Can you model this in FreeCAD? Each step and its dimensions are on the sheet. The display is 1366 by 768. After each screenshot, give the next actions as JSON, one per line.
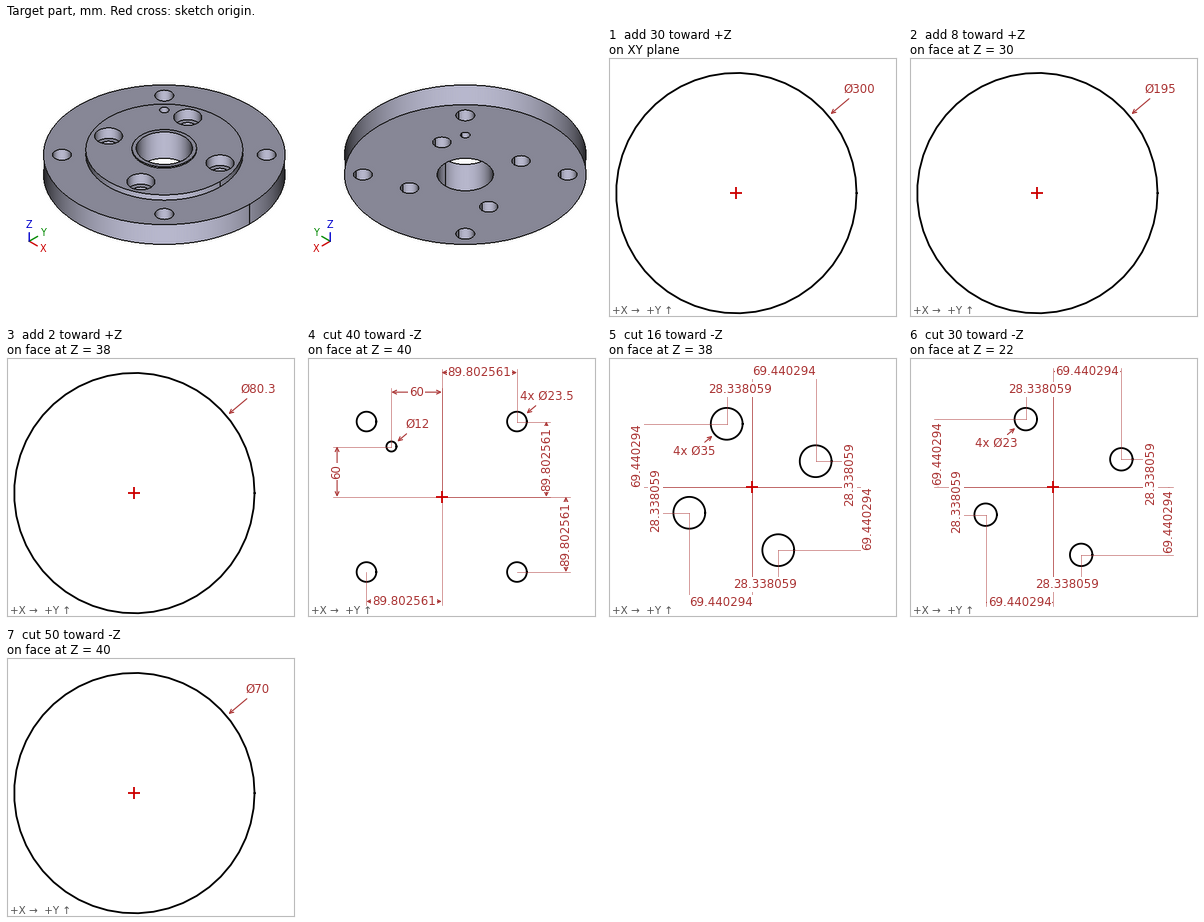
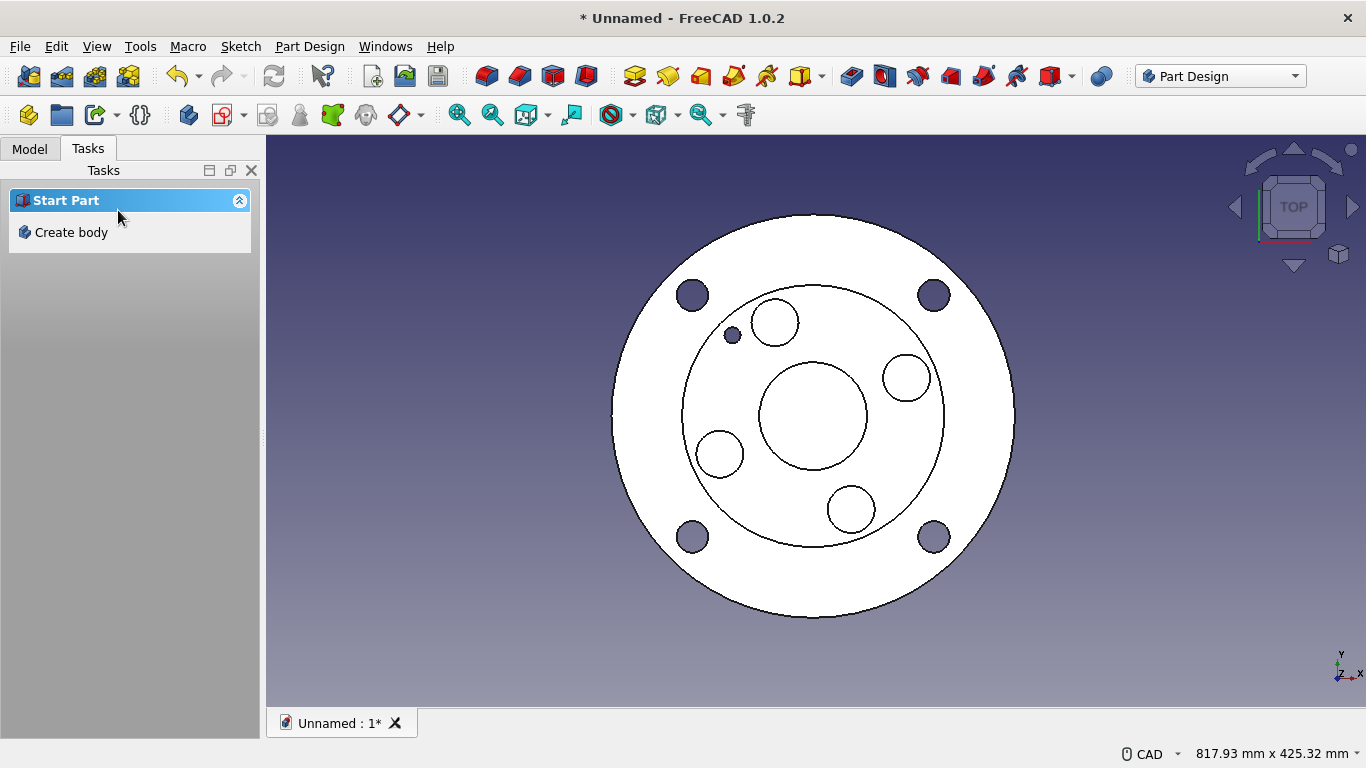
{"action": "left_click", "coordinate": [720, 453]}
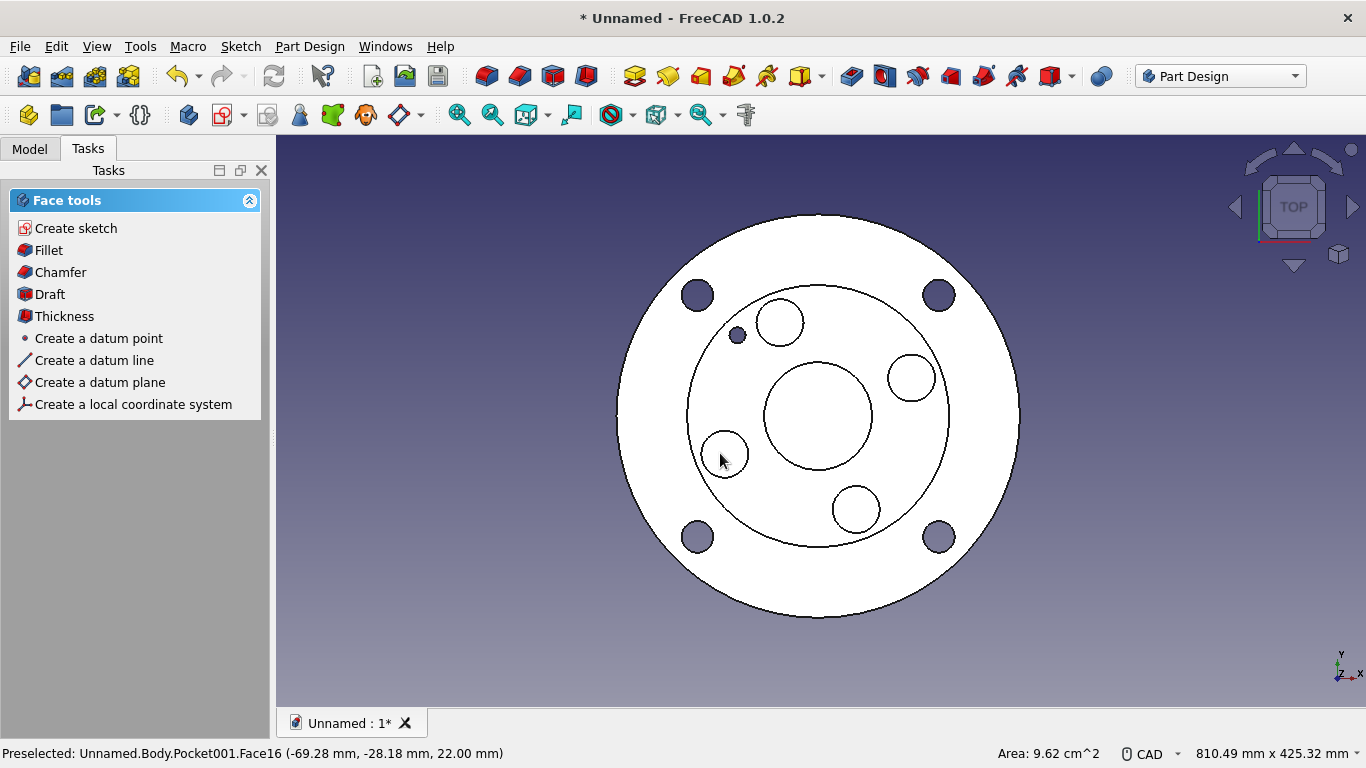
{"action": "left_click", "coordinate": [222, 116]}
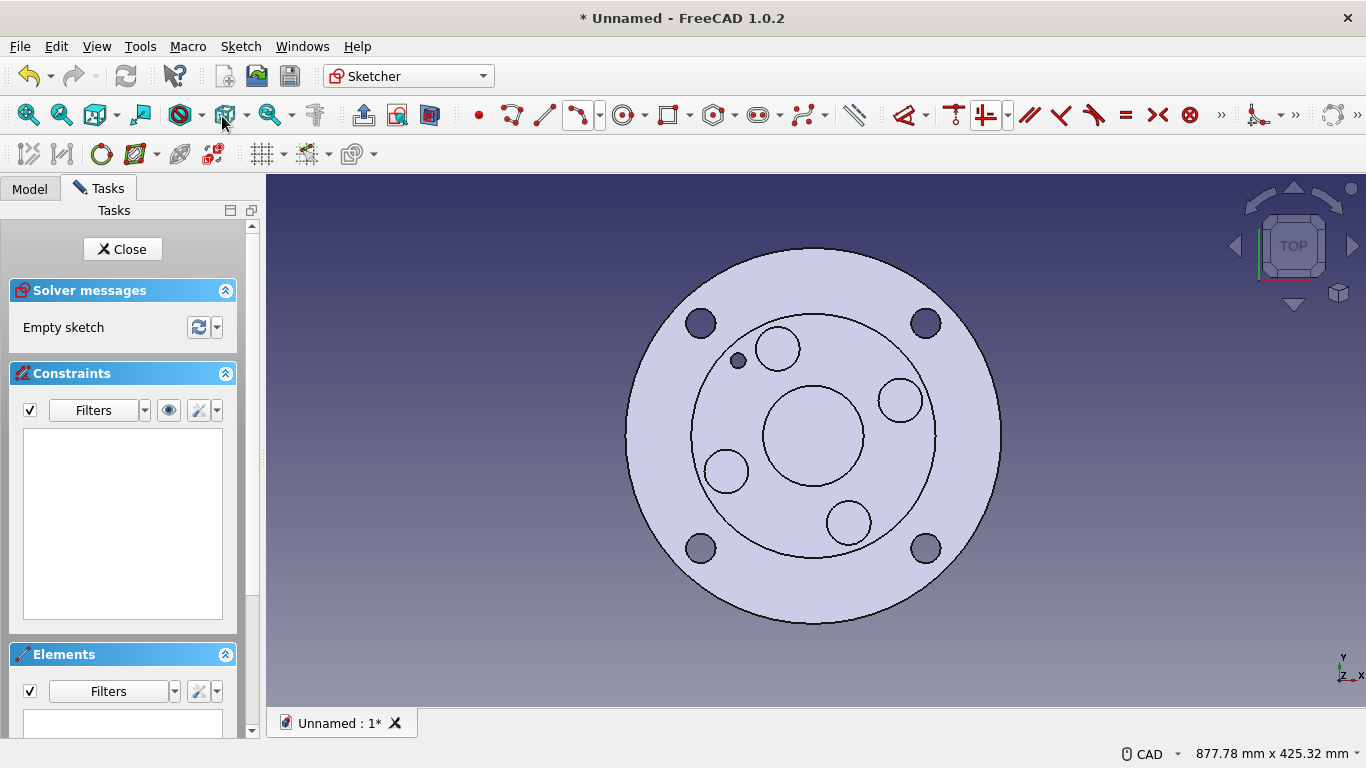
{"action": "scroll", "coordinate": [893, 430], "scroll_direction": "up", "scroll_amount": 3}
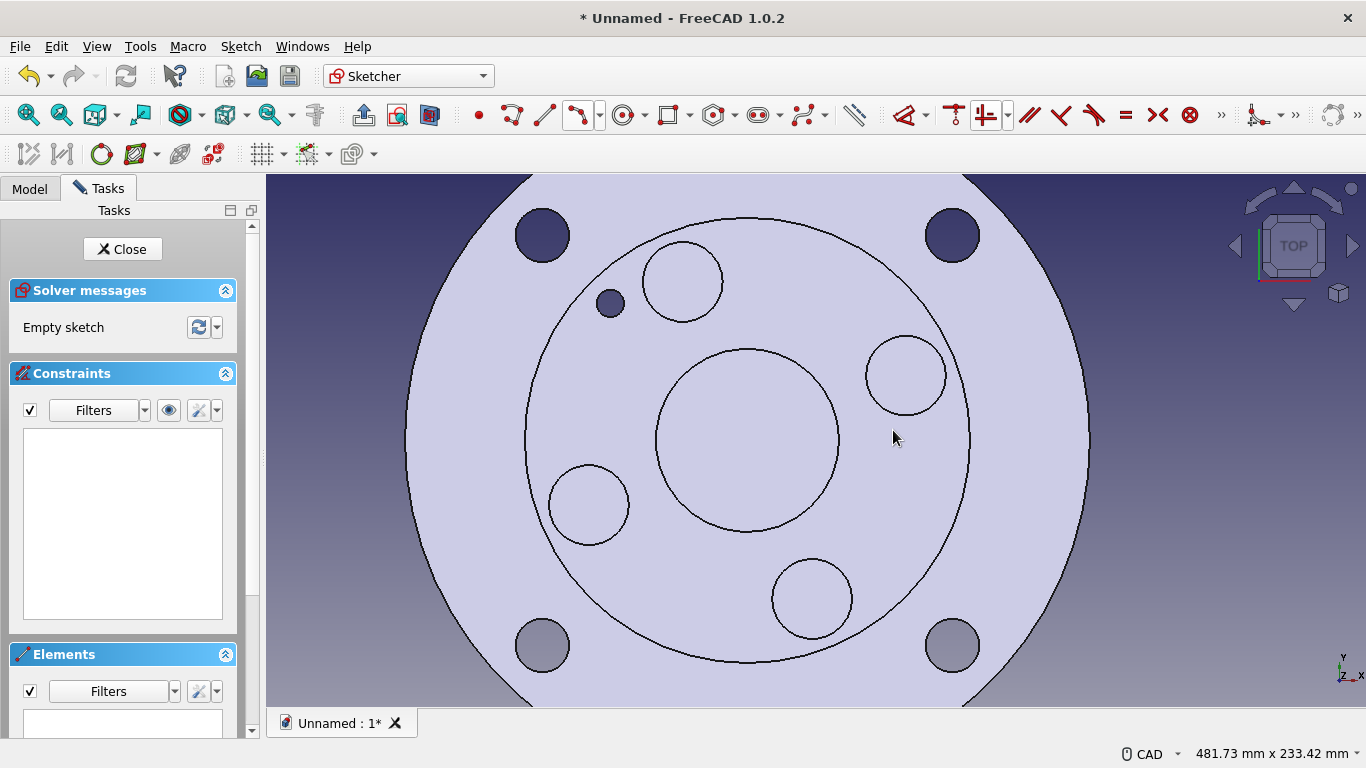
{"action": "left_click", "coordinate": [622, 116]}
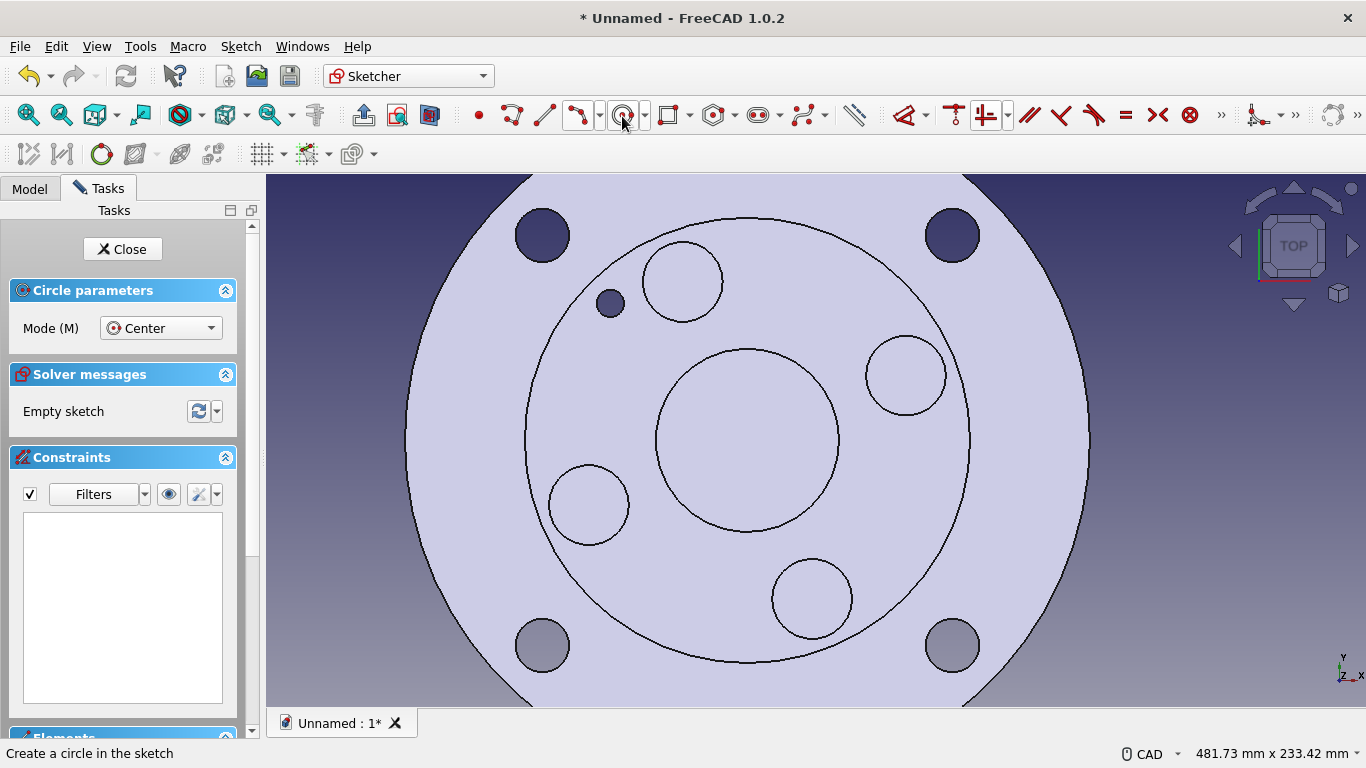
{"action": "left_click", "coordinate": [683, 282]}
{"action": "left_click", "coordinate": [701, 263]}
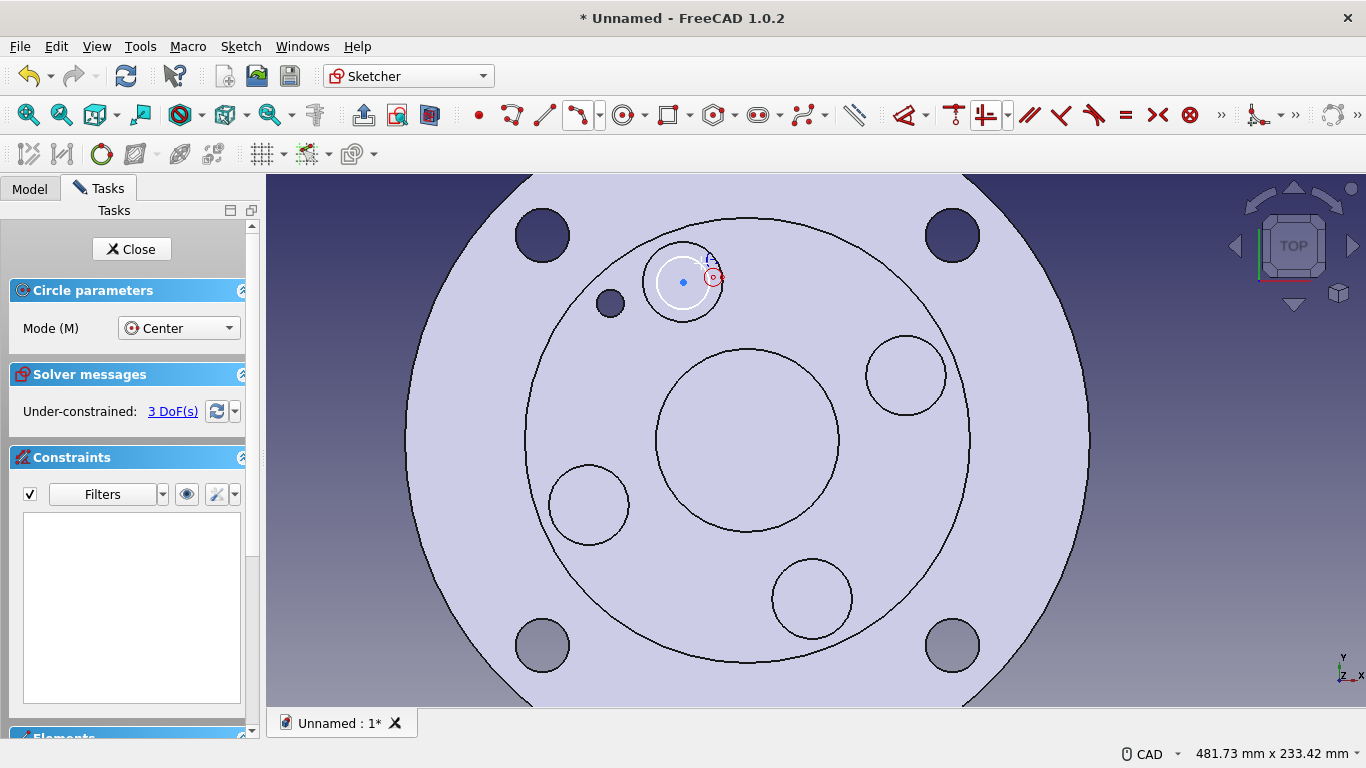
{"action": "left_click", "coordinate": [906, 376]}
{"action": "left_click", "coordinate": [925, 357]}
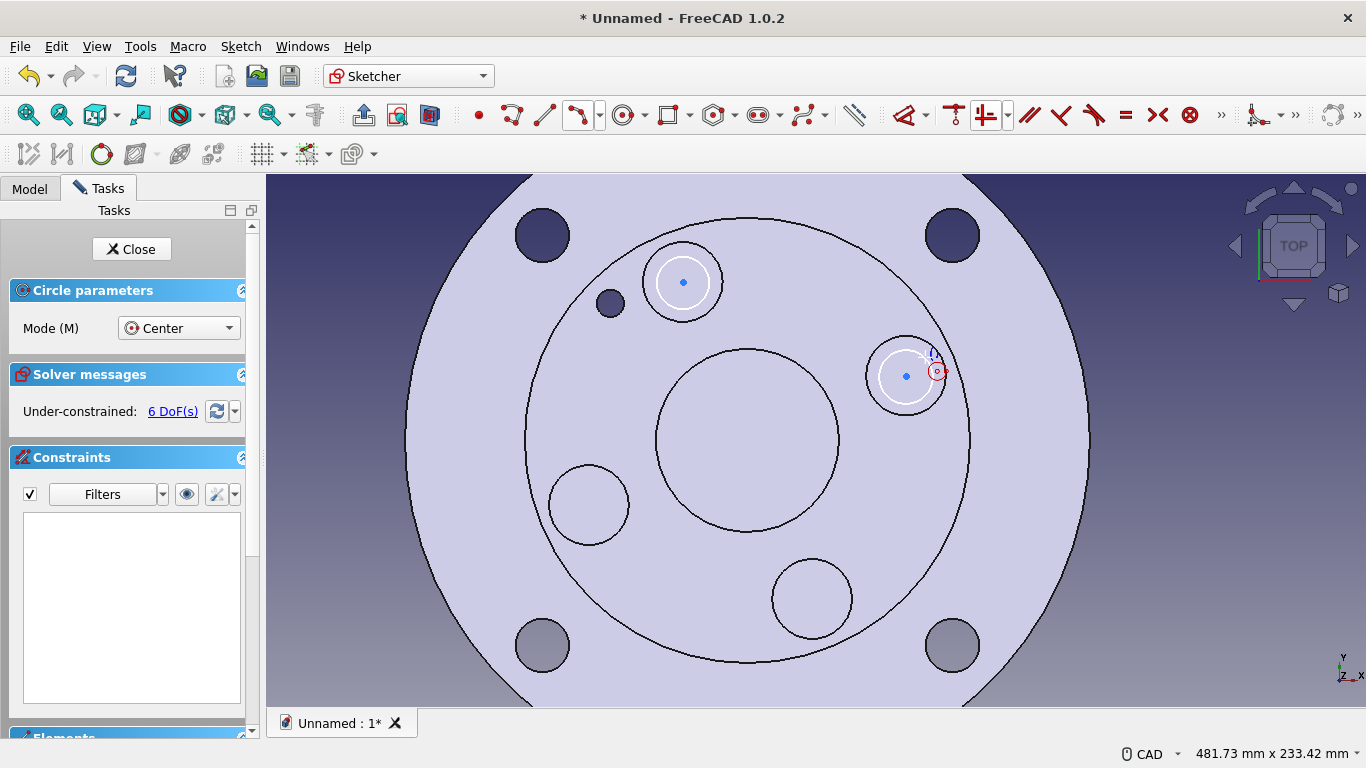
{"action": "left_click", "coordinate": [812, 599]}
{"action": "left_click", "coordinate": [831, 580]}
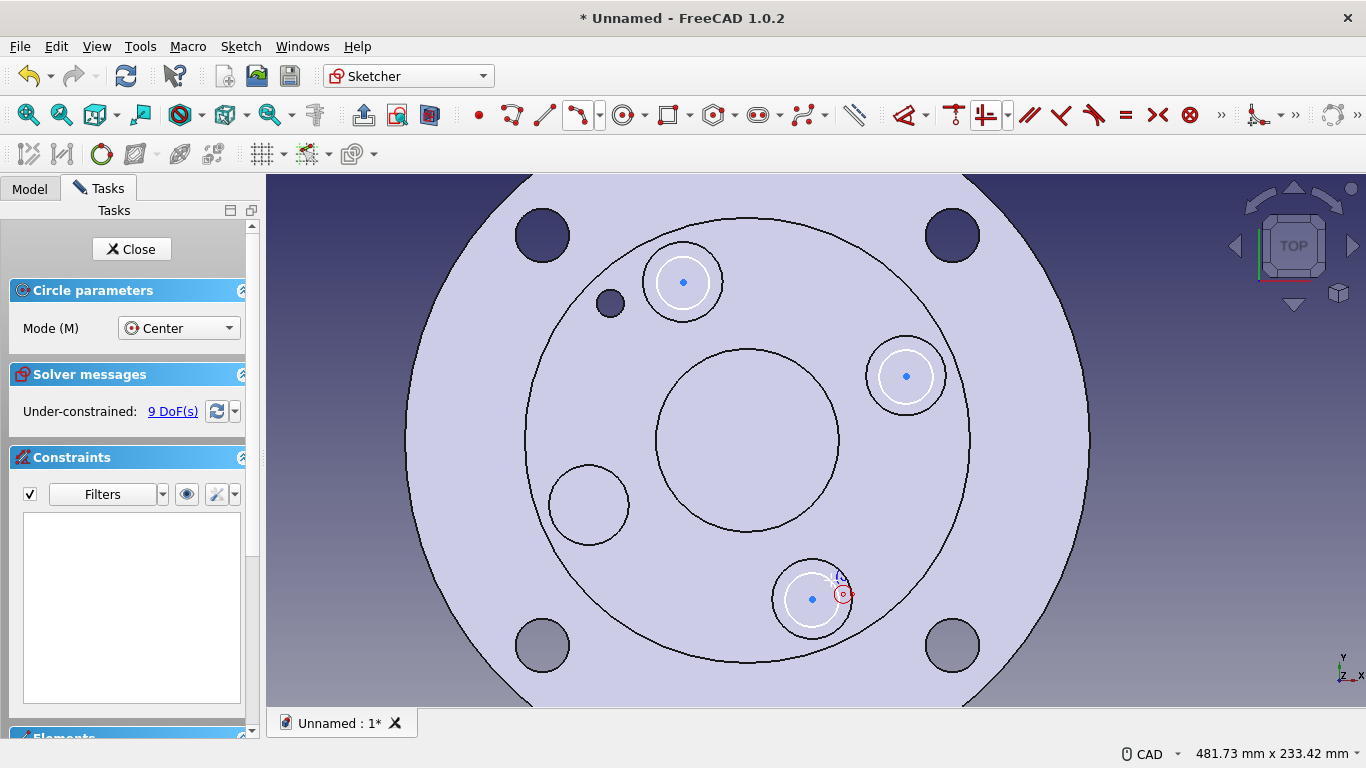
{"action": "left_click", "coordinate": [589, 505]}
{"action": "left_click", "coordinate": [607, 487]}
{"action": "key", "text": "Escape"}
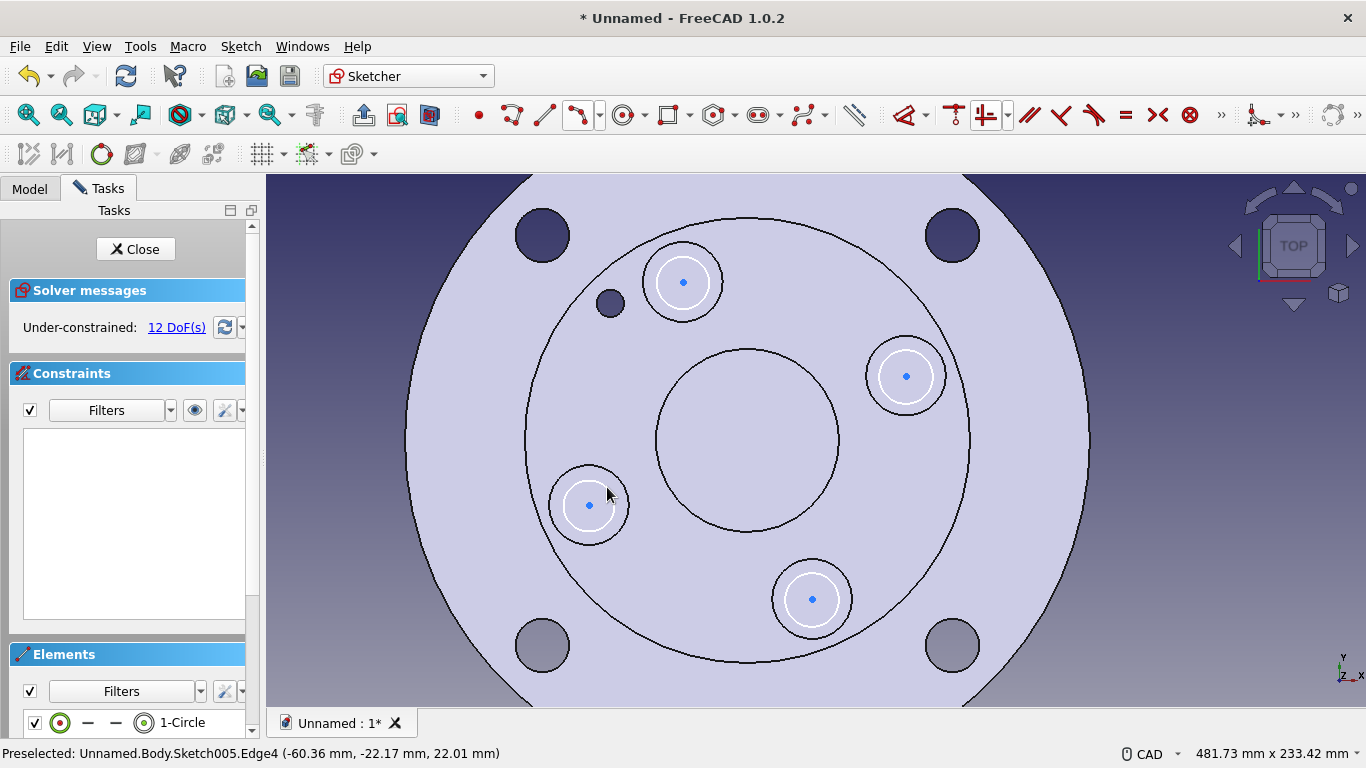
{"action": "left_click", "coordinate": [701, 264]}